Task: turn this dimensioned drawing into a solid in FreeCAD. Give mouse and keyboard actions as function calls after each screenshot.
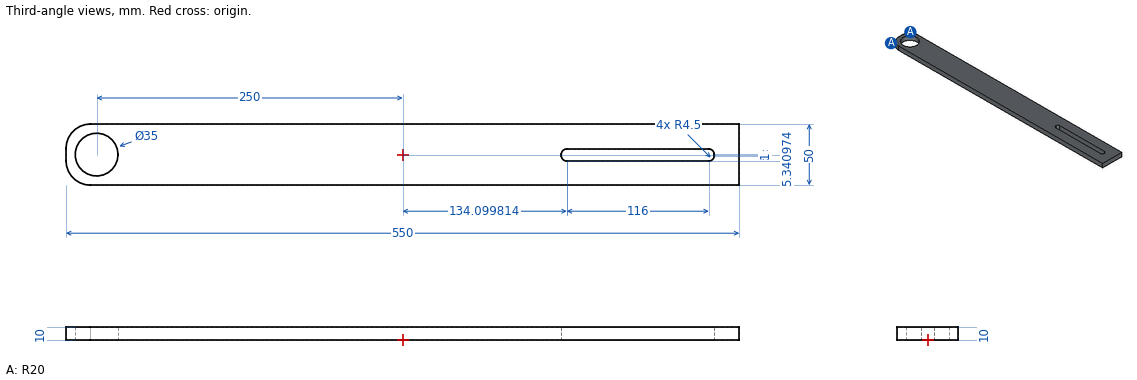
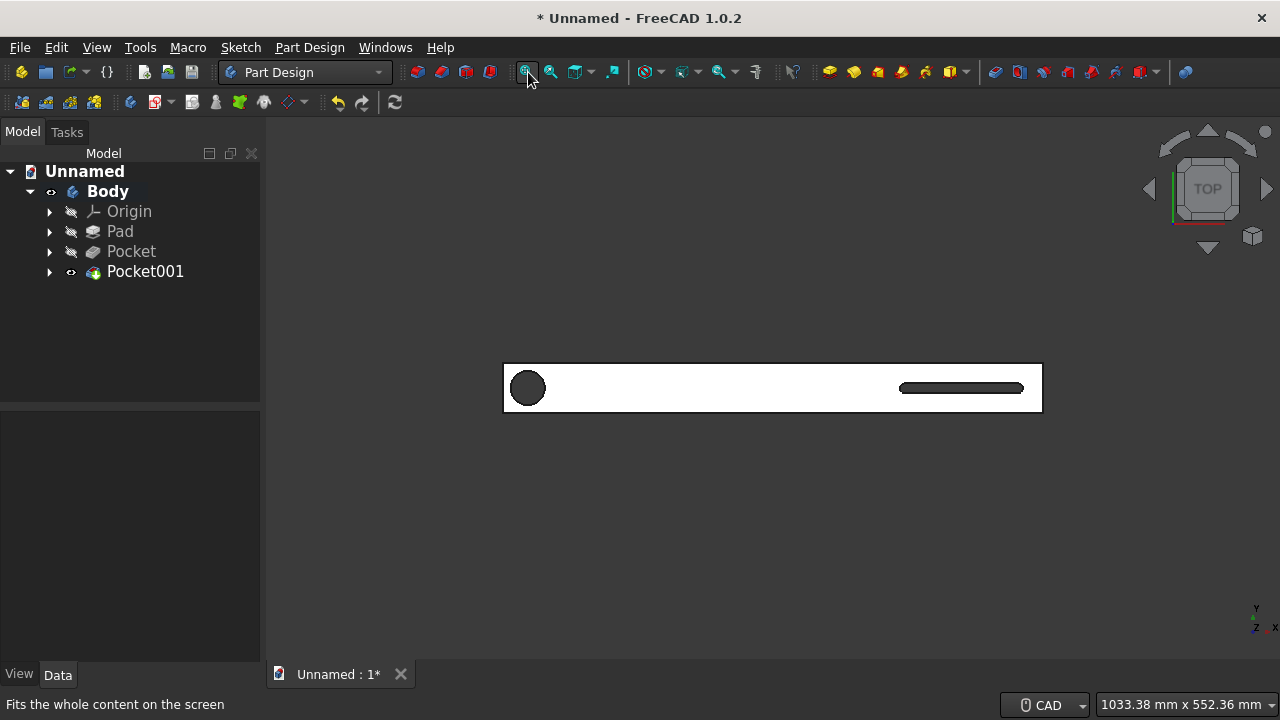
key(1)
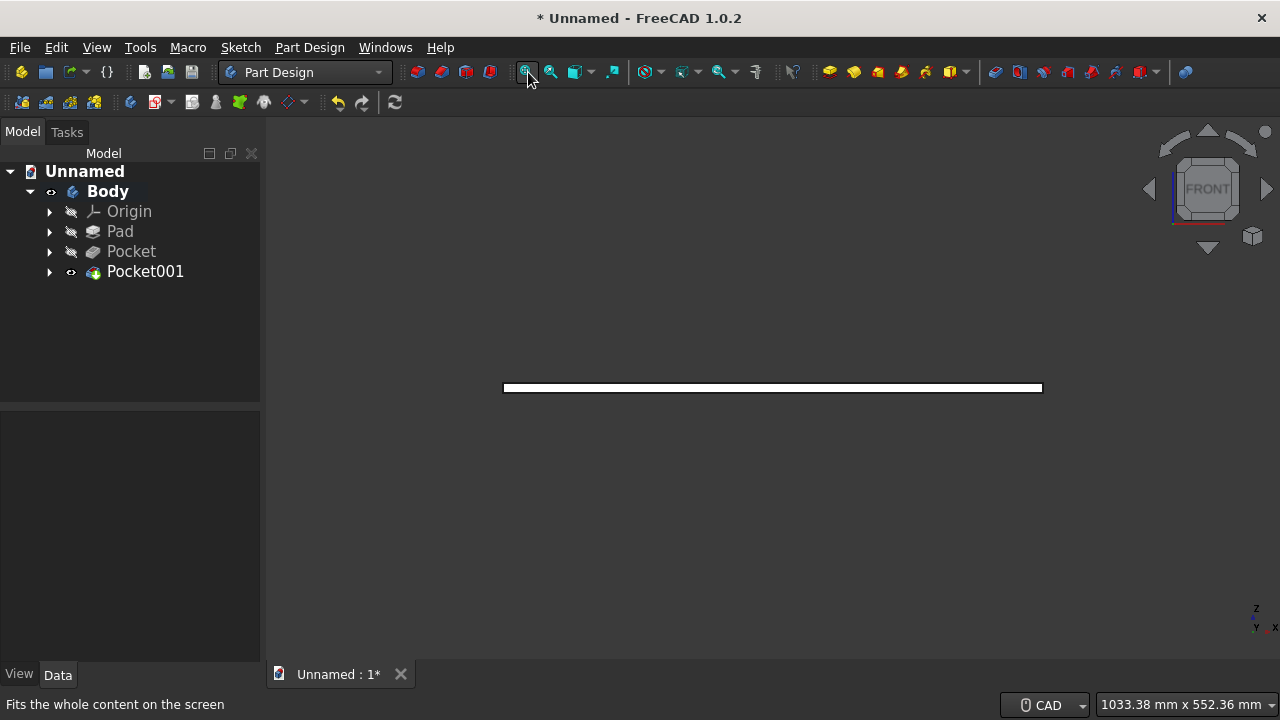
scroll(503, 387, up, 8)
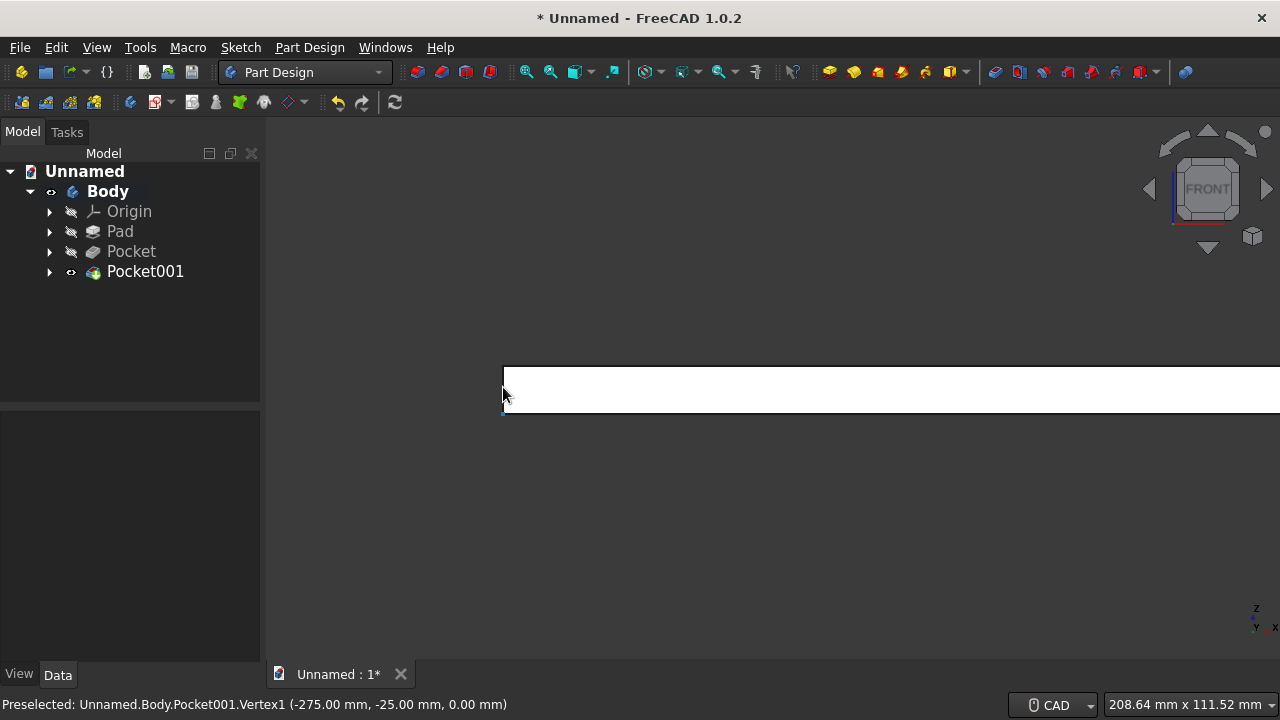
click(503, 389)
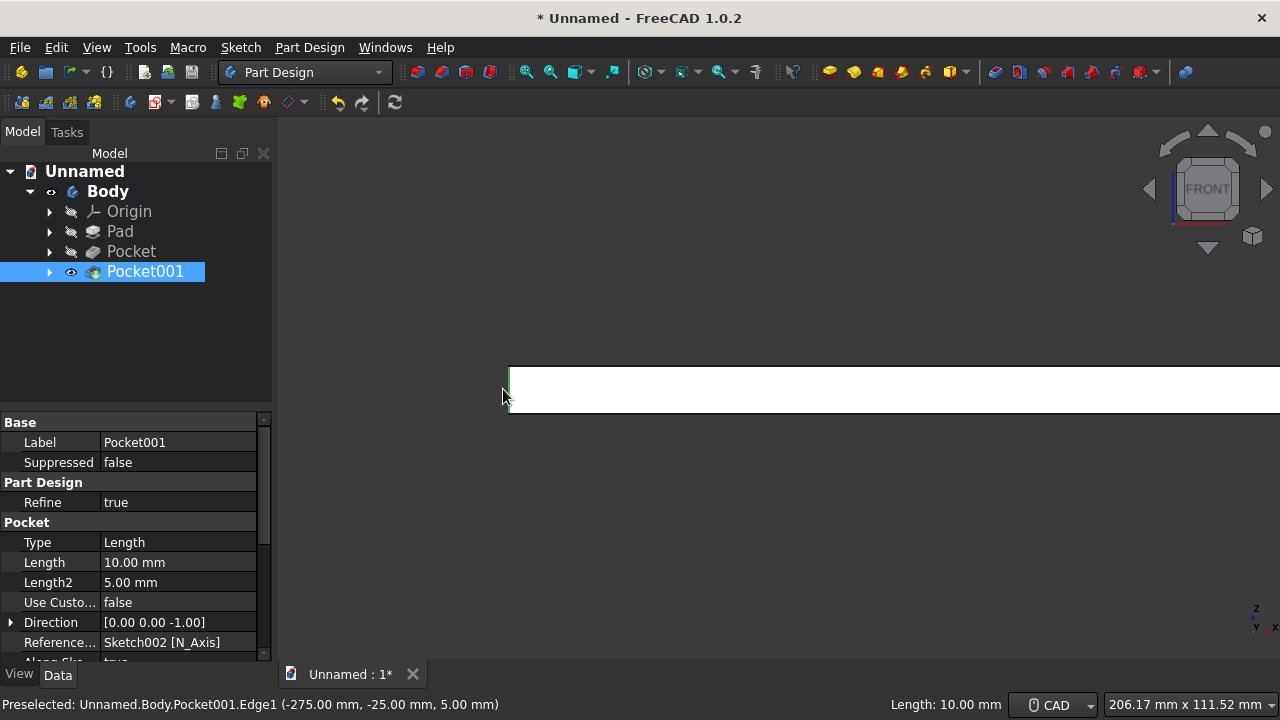
click(528, 72)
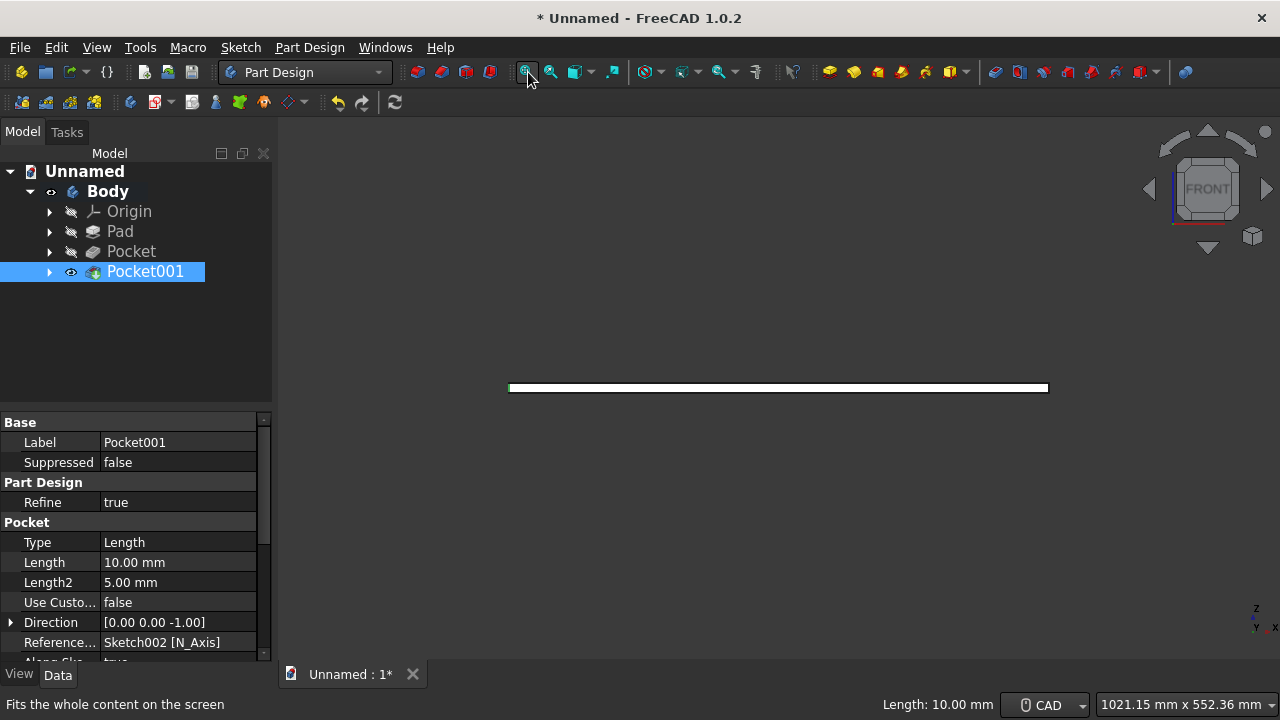
key(3)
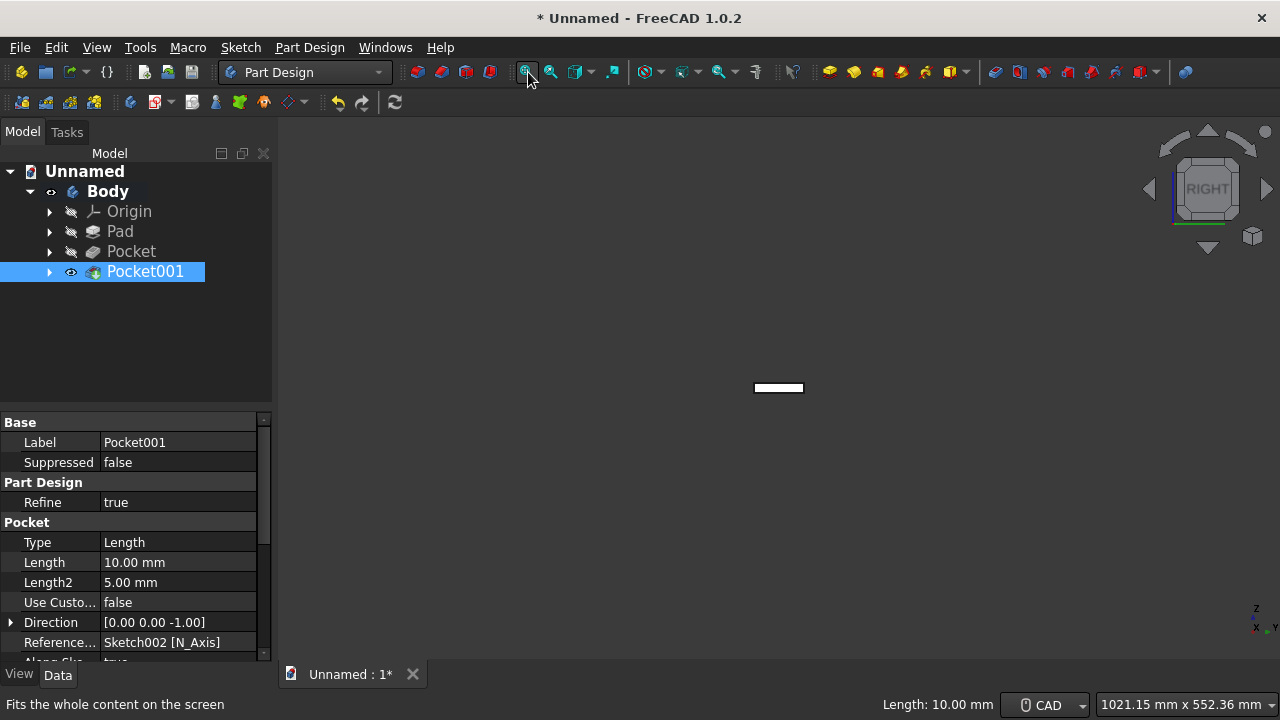
click(528, 72)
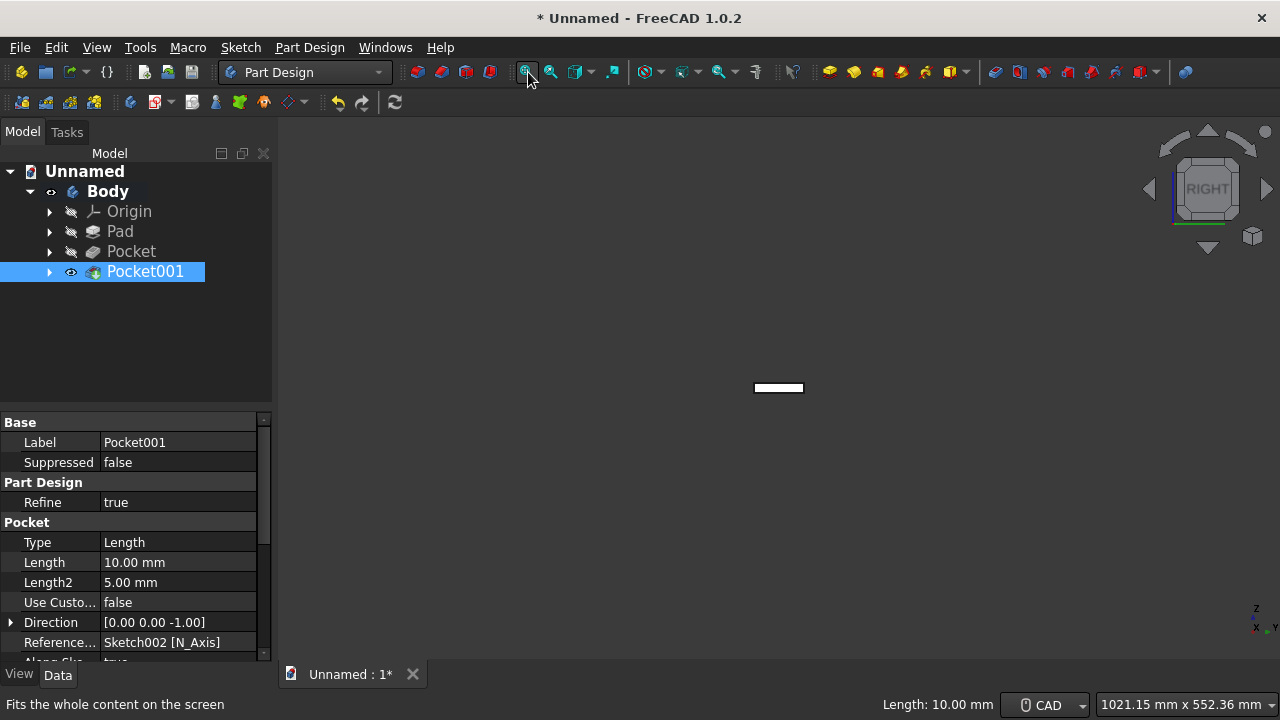
scroll(804, 387, up, 8)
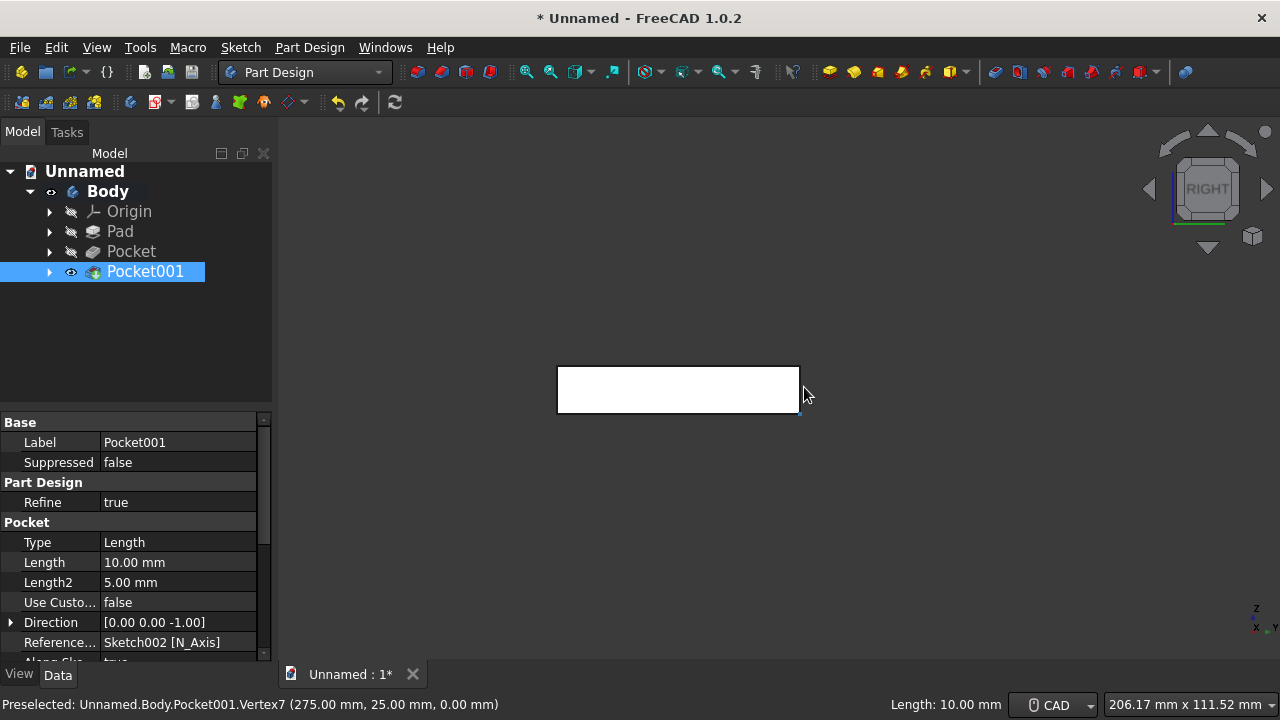
key(v)
key(f)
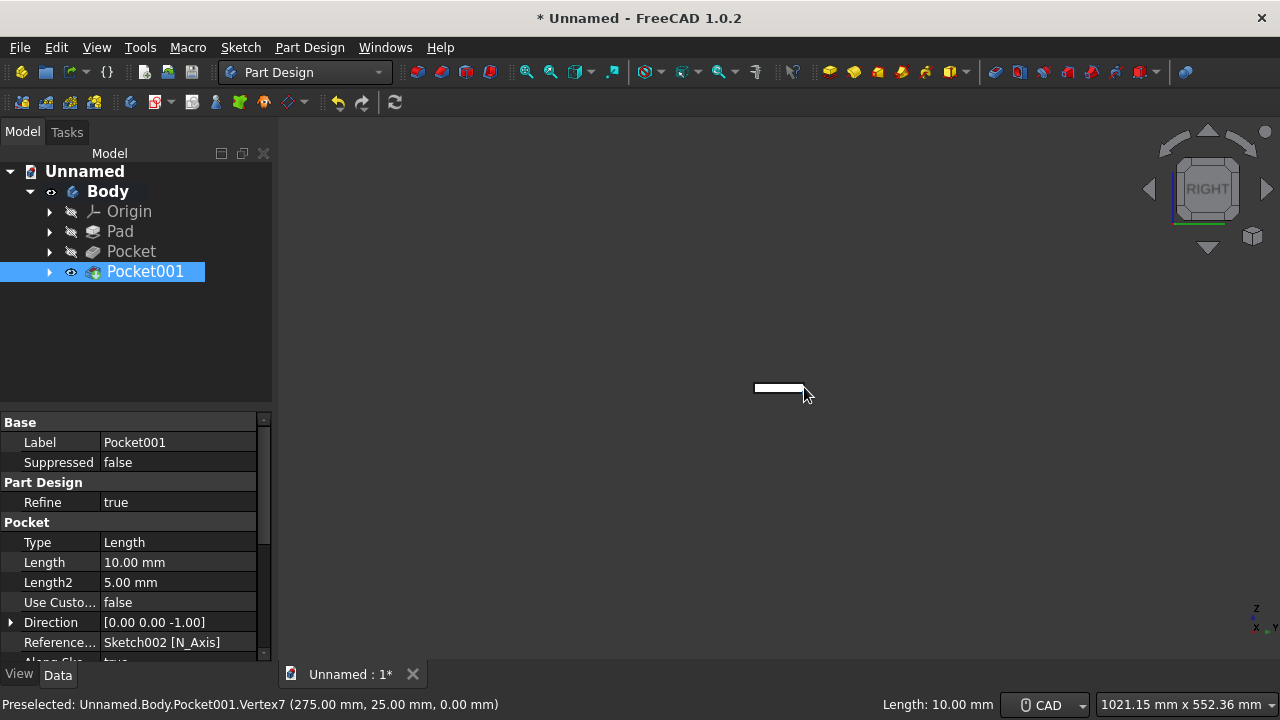
key(5)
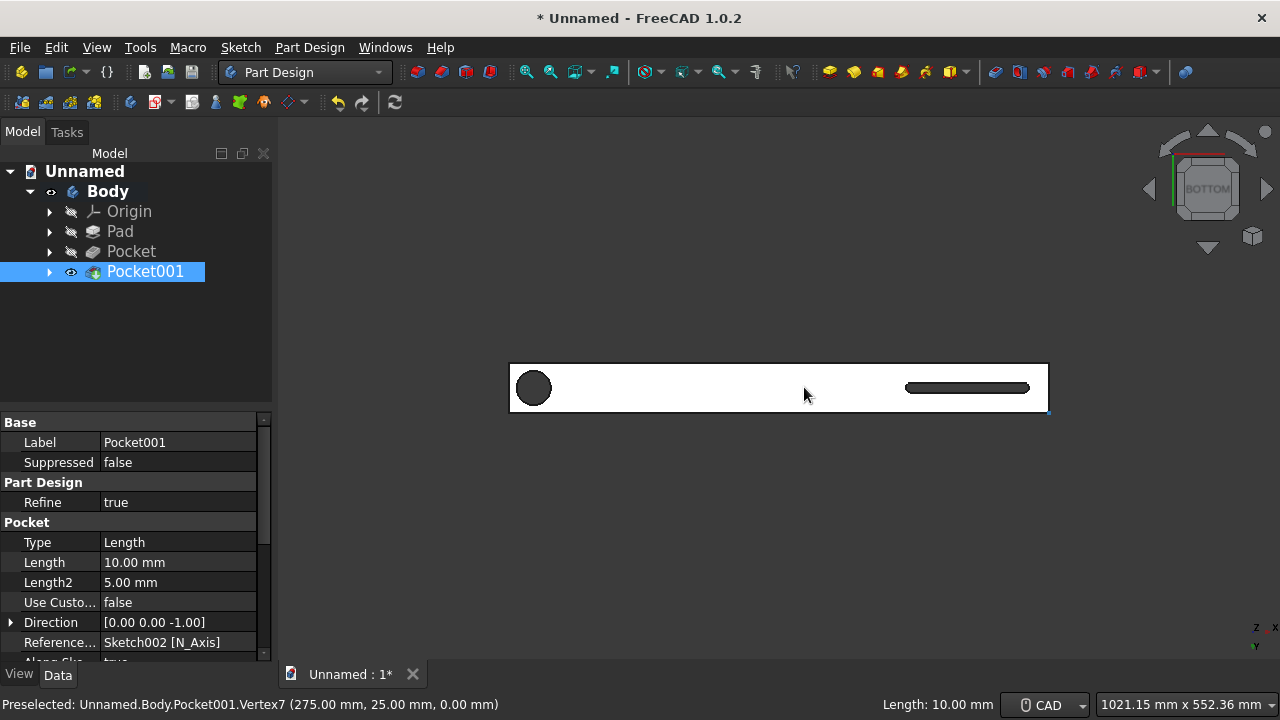
scroll(509, 412, up, 8)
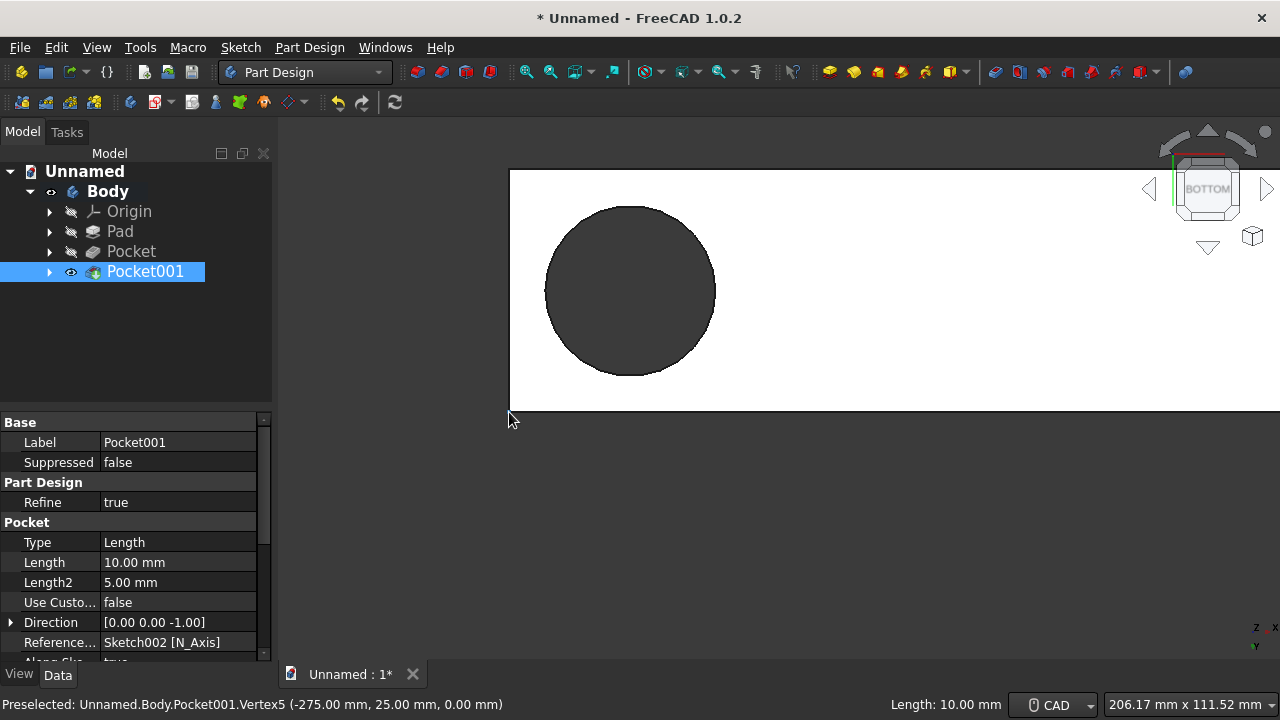
click(528, 72)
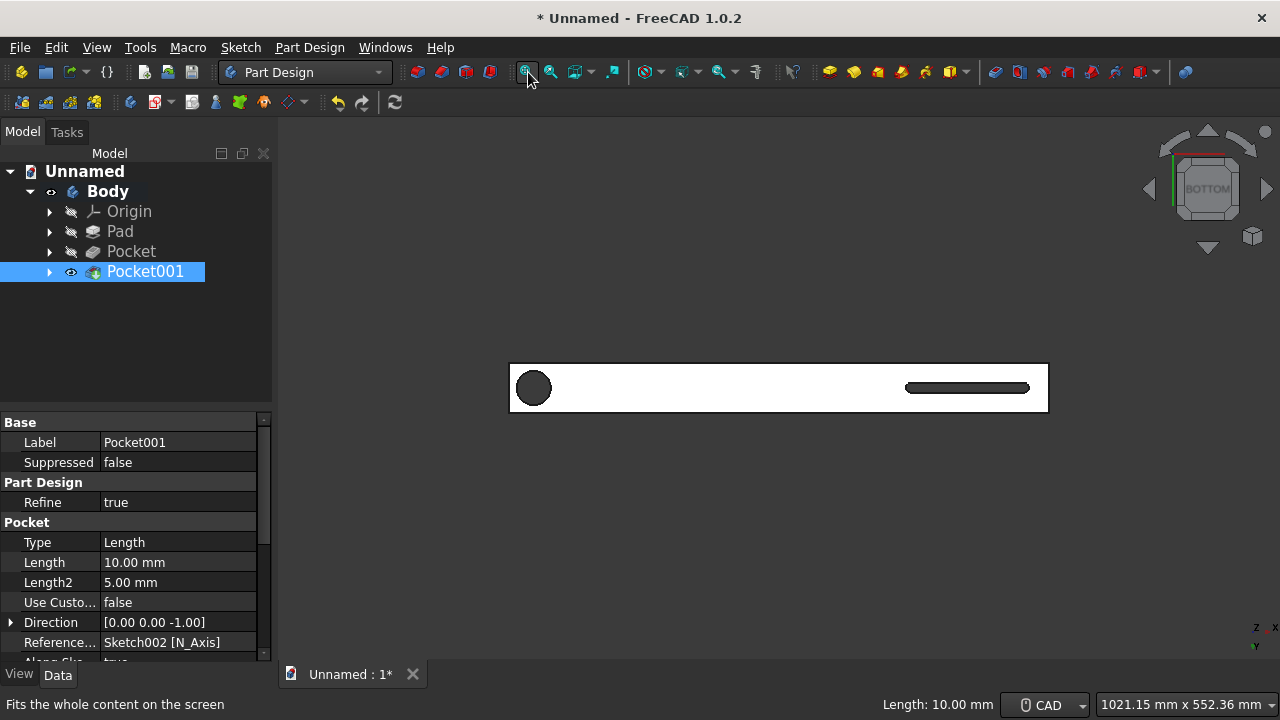
key(4)